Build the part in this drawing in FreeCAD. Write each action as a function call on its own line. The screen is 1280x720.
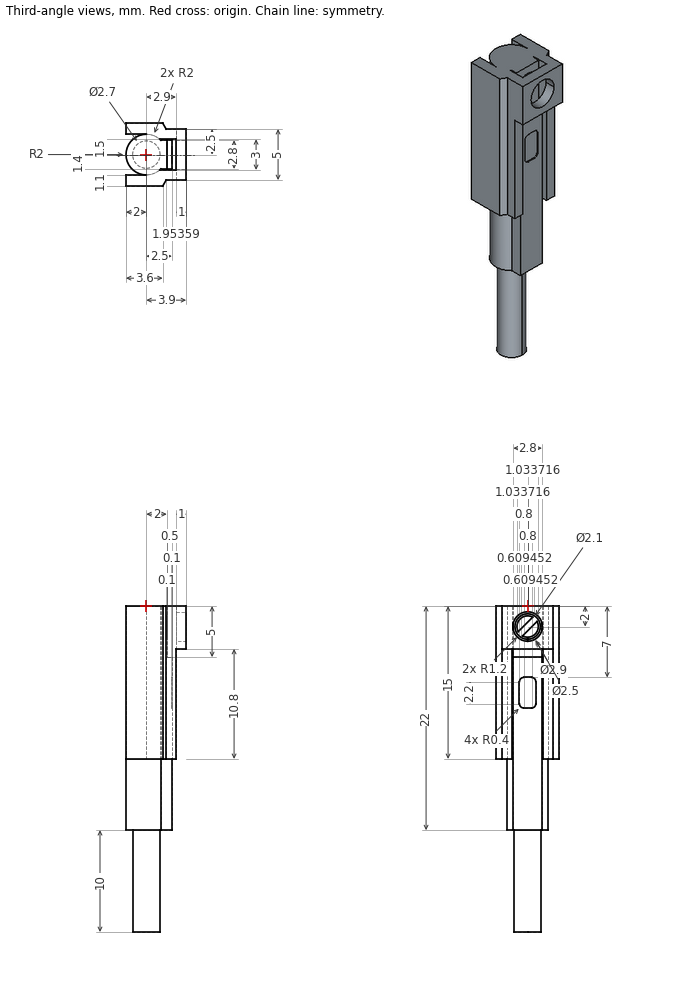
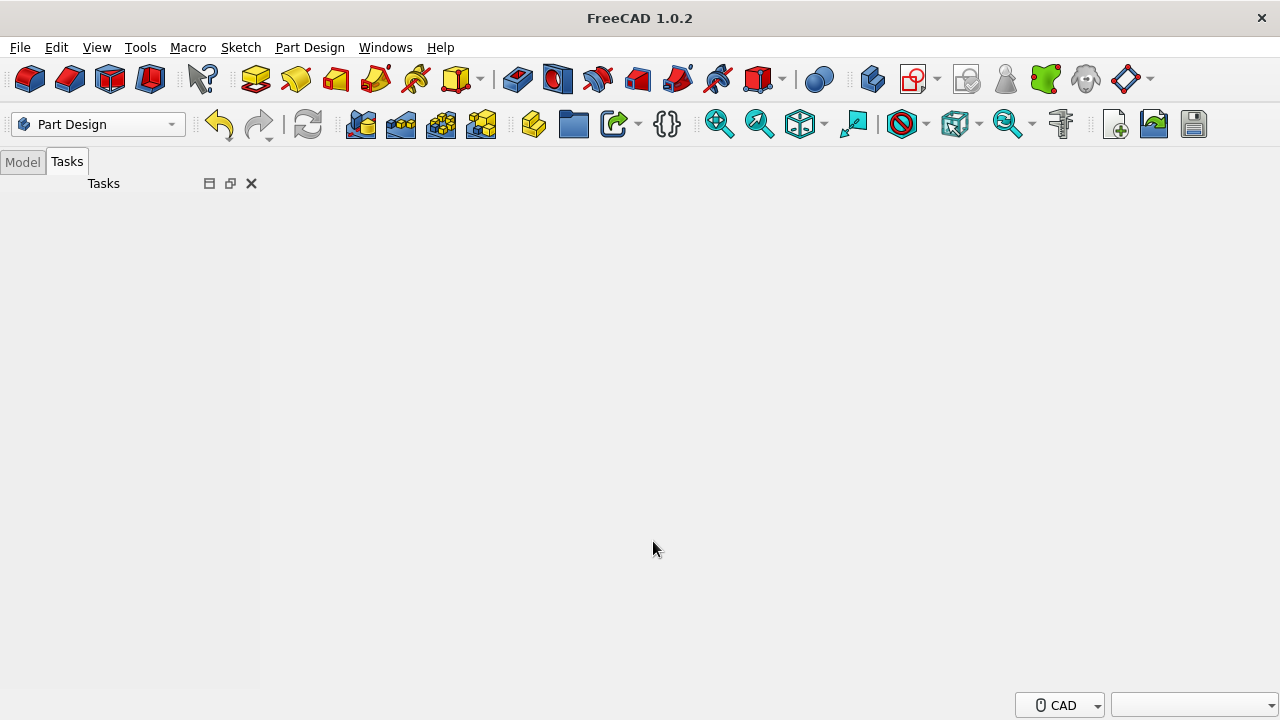
click(1114, 124)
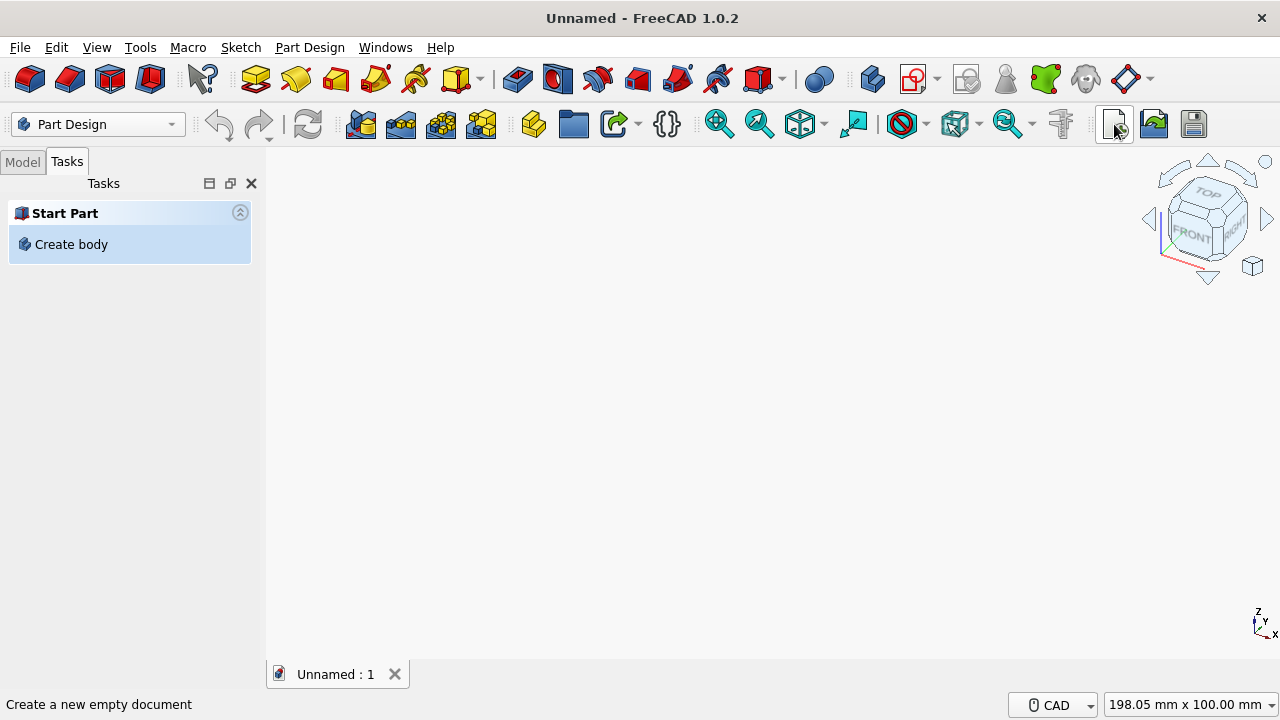
click(914, 80)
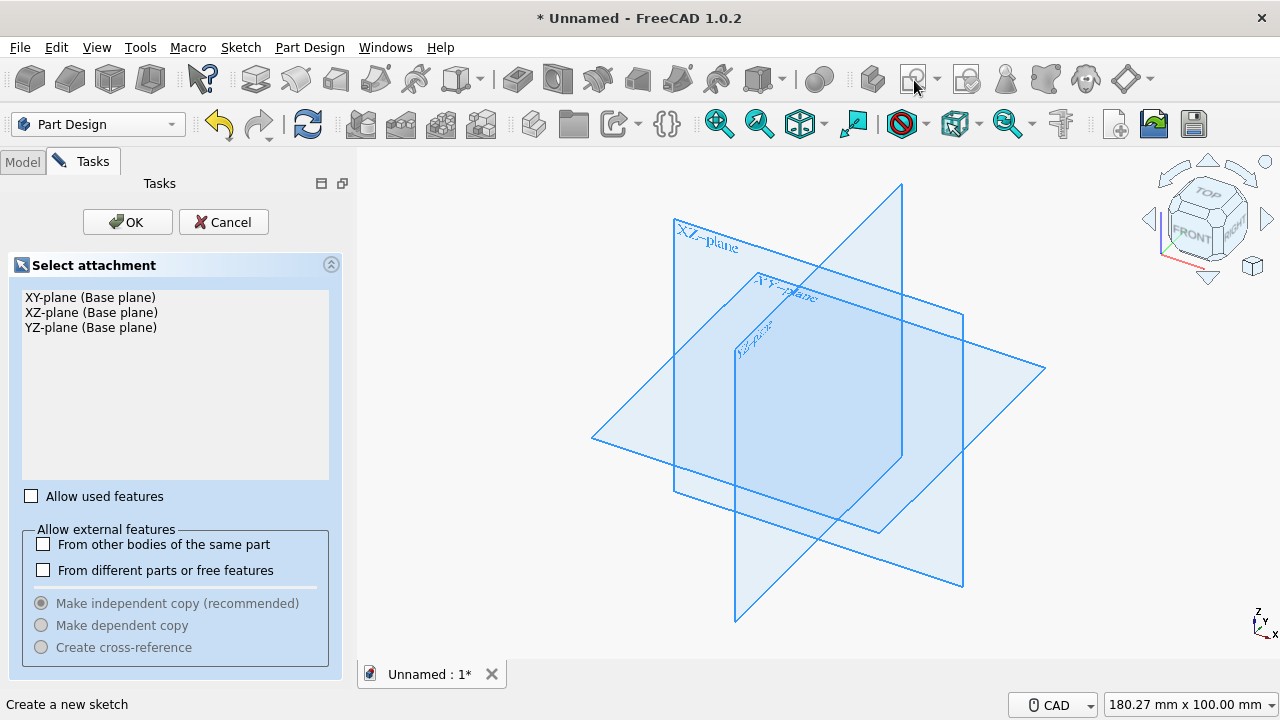
click(82, 298)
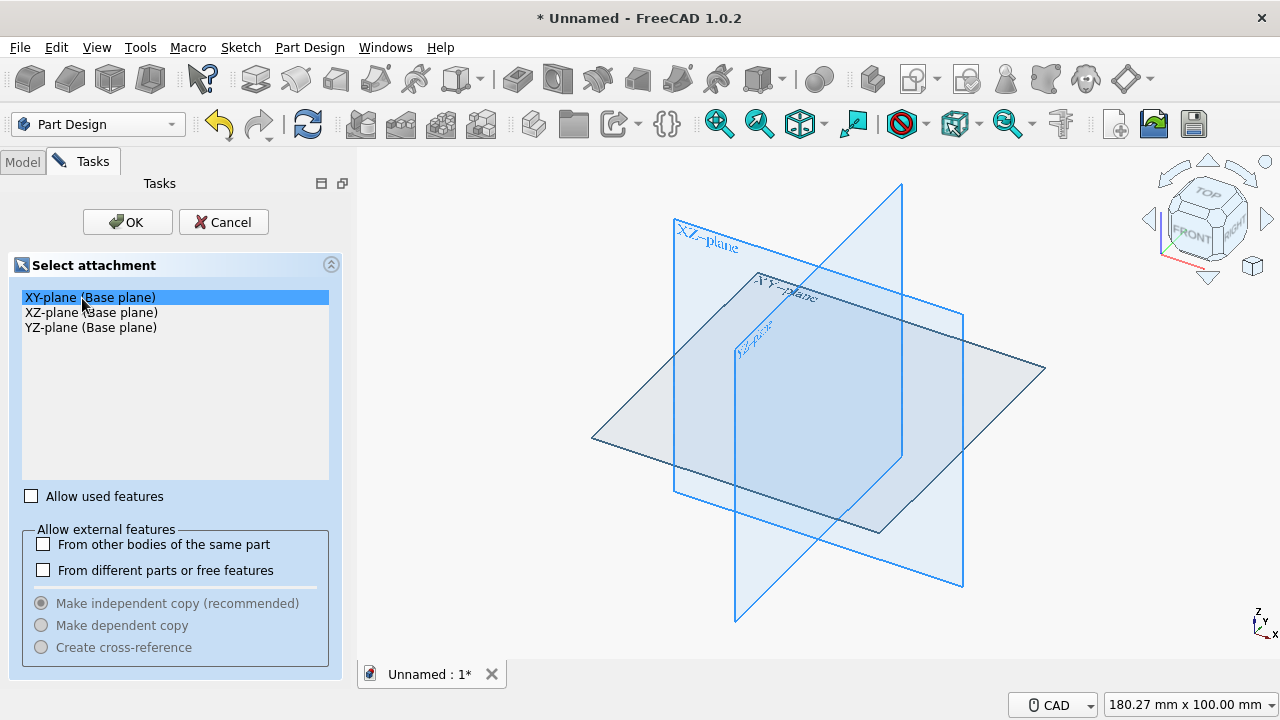
click(128, 222)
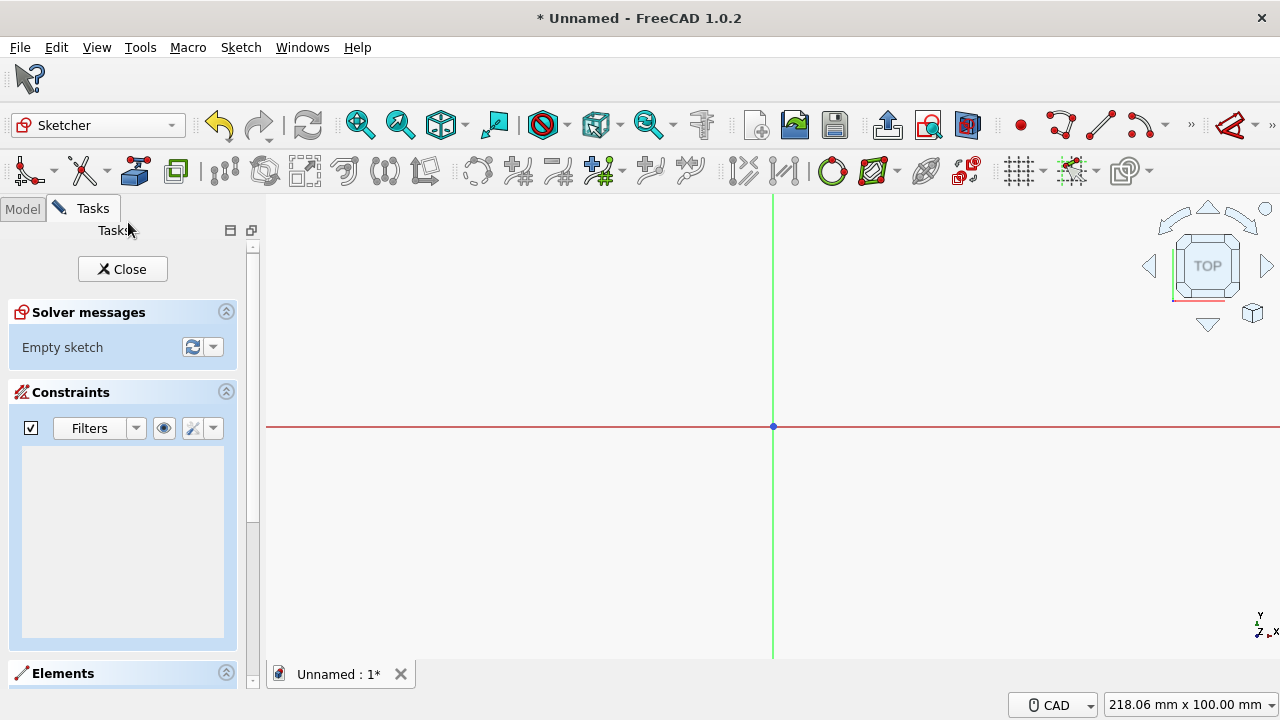
scroll(785, 426, up, 12)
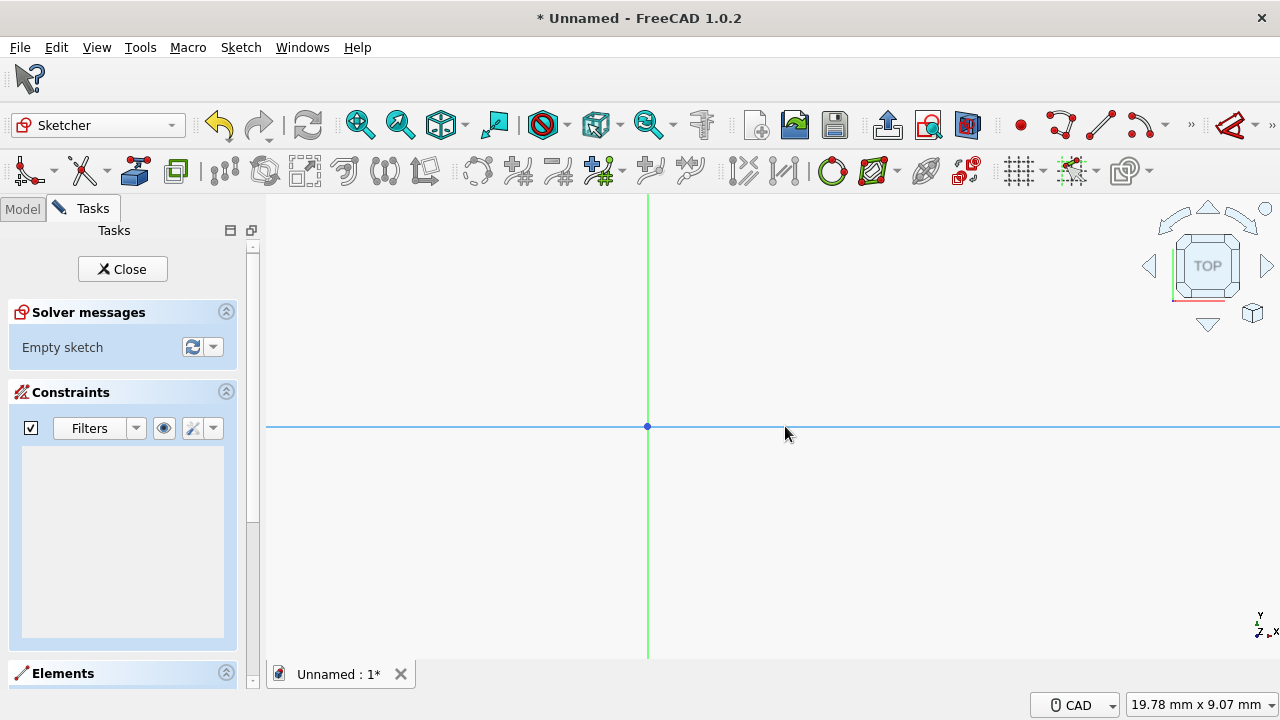
click(1062, 126)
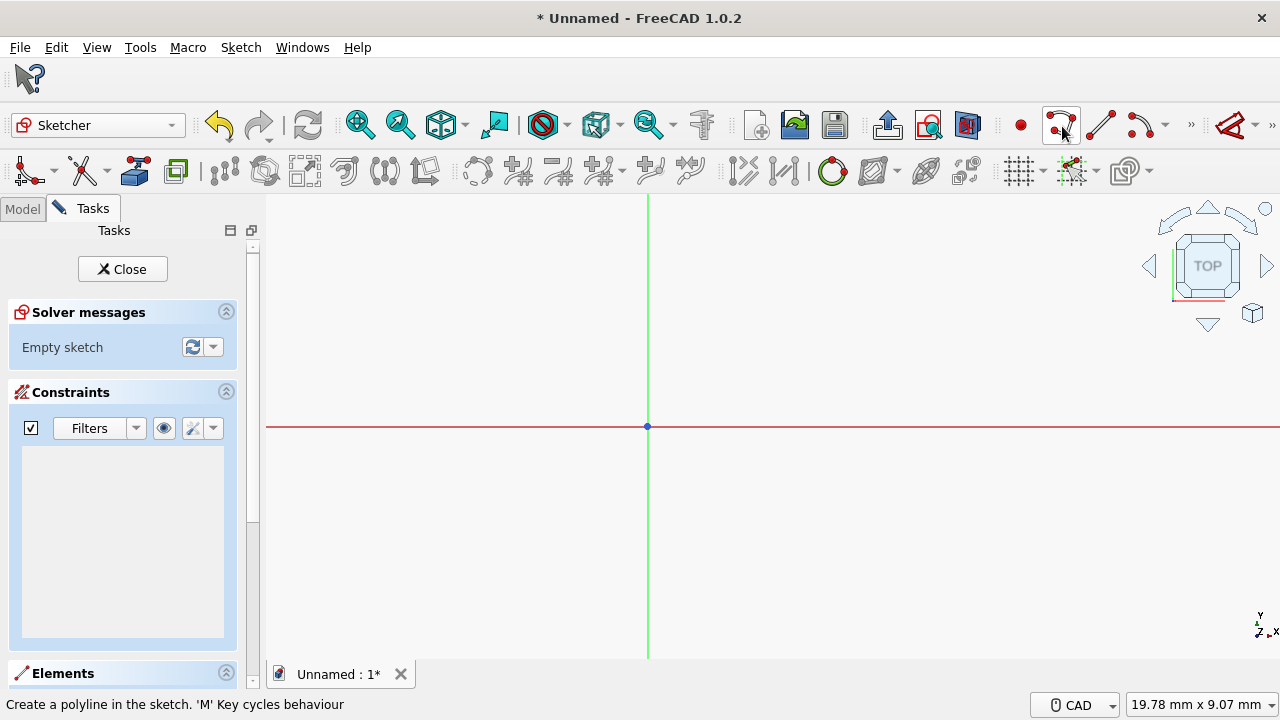
click(715, 350)
click(796, 350)
click(796, 503)
click(715, 503)
right_click(715, 503)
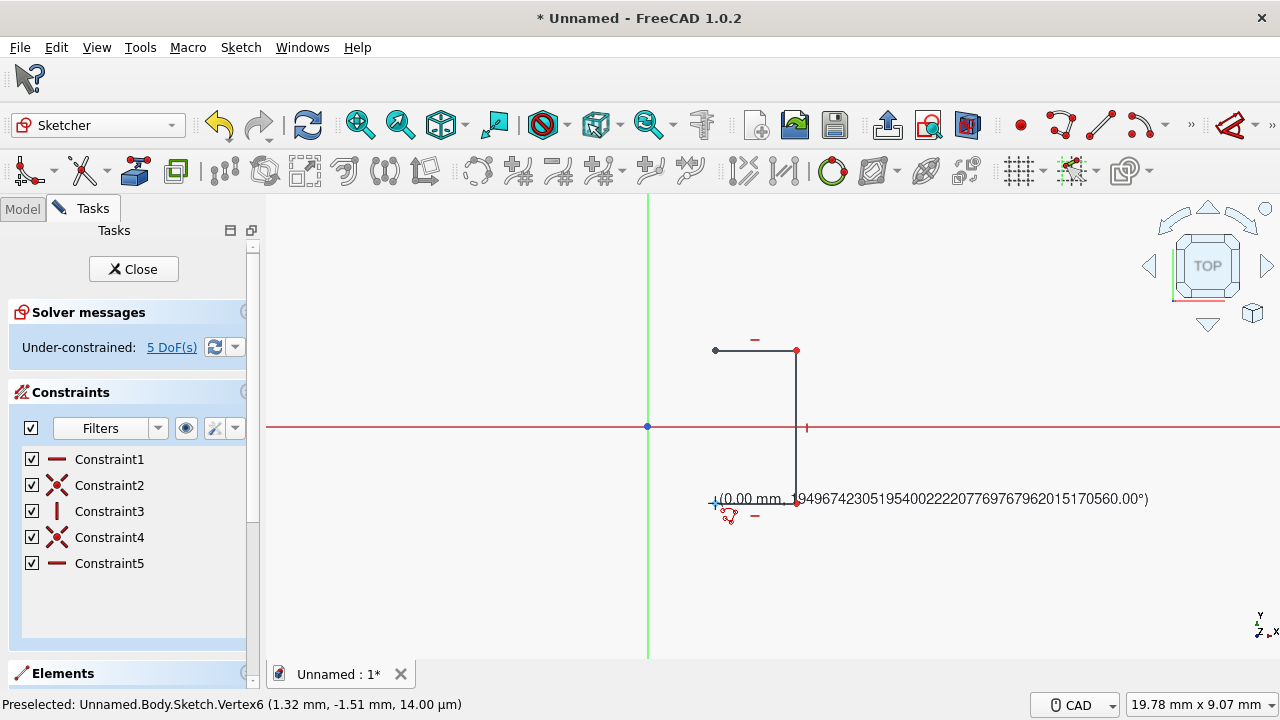
click(648, 529)
click(545, 529)
click(545, 585)
click(730, 585)
click(747, 555)
click(847, 555)
click(847, 298)
click(747, 298)
click(730, 268)
click(545, 268)
click(545, 324)
click(648, 324)
right_click(648, 324)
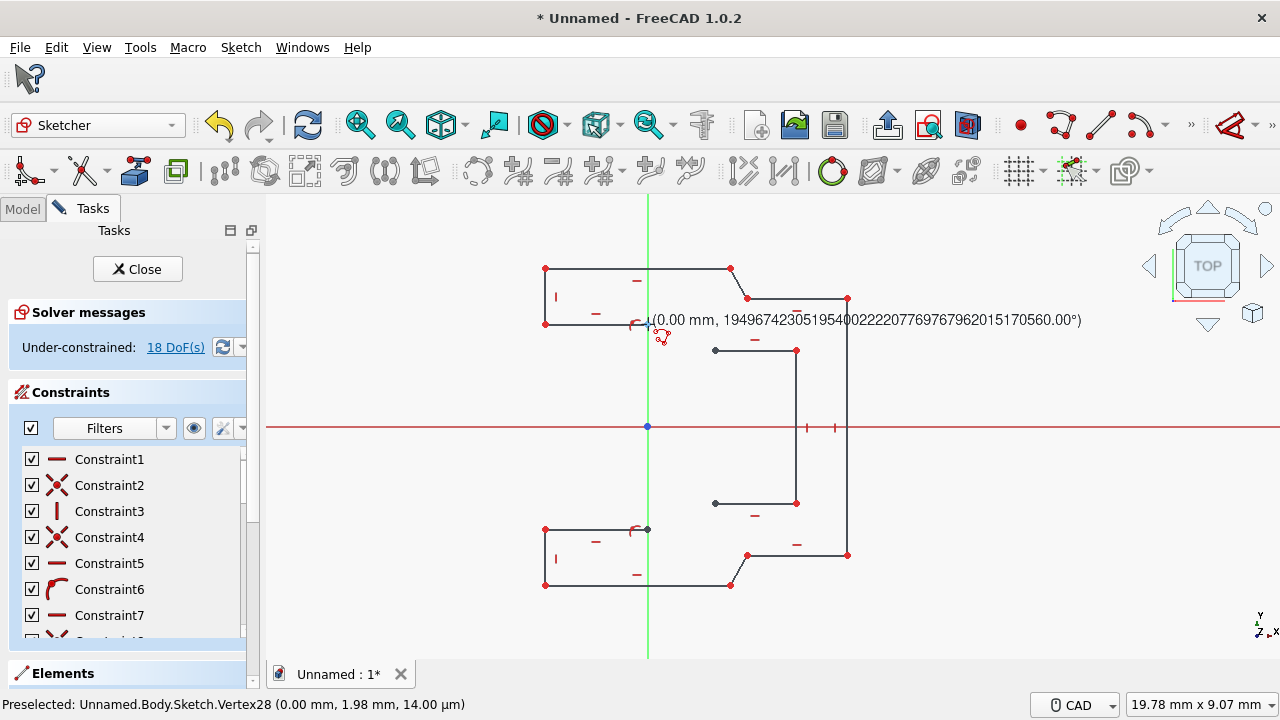
click(1168, 126)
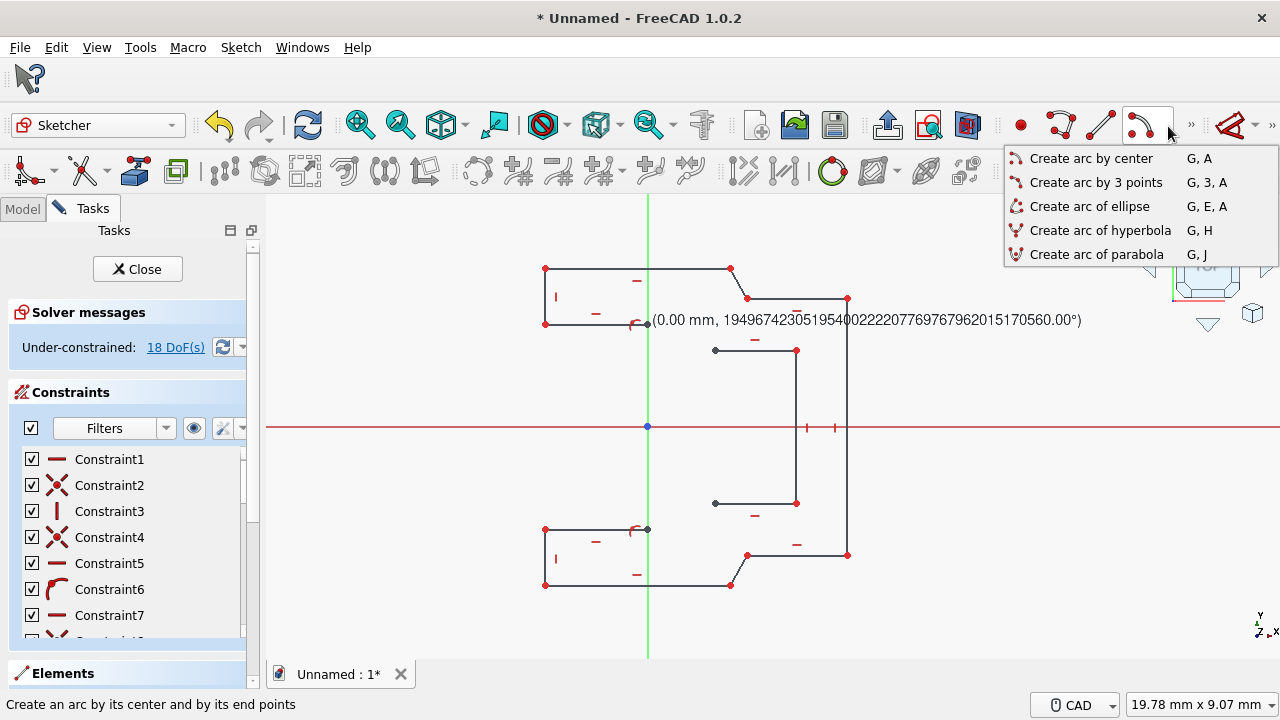
click(1142, 182)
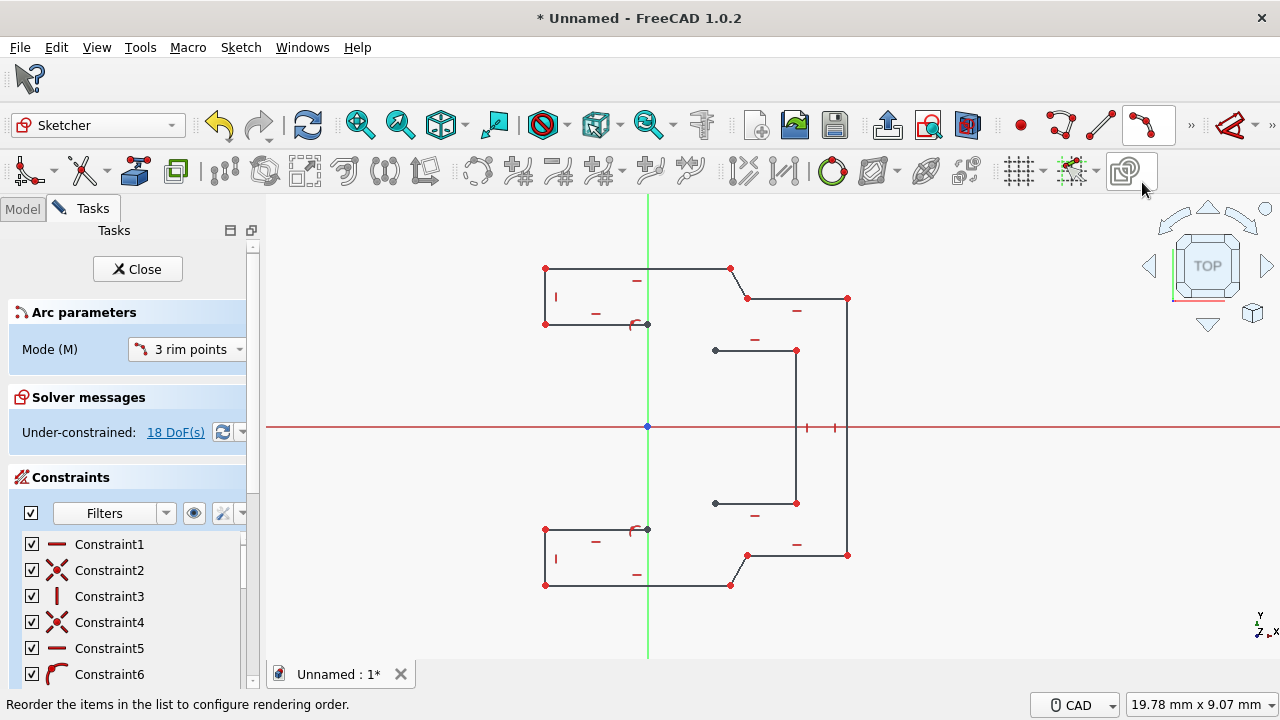
click(715, 504)
click(648, 530)